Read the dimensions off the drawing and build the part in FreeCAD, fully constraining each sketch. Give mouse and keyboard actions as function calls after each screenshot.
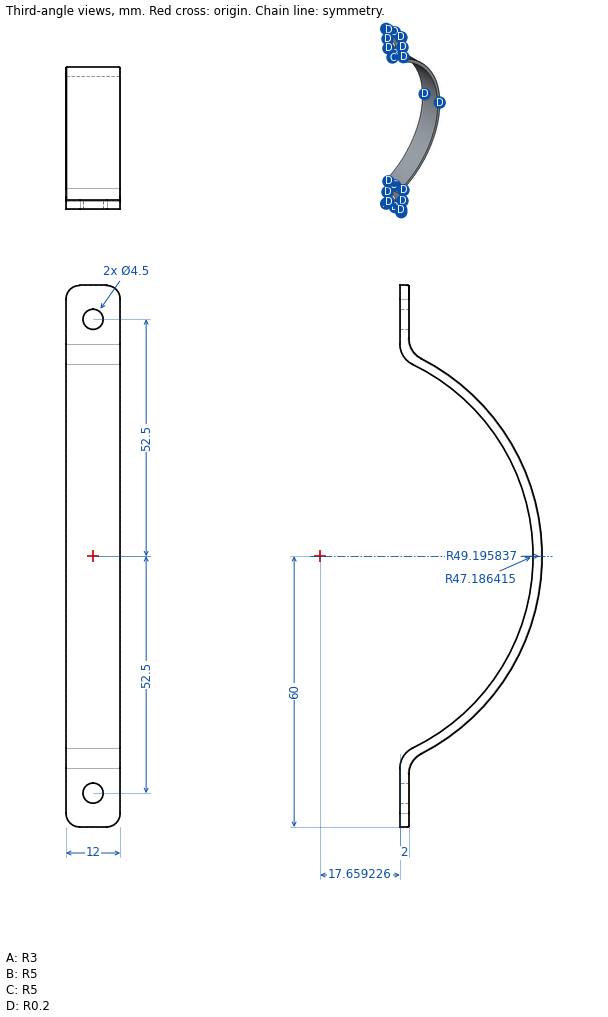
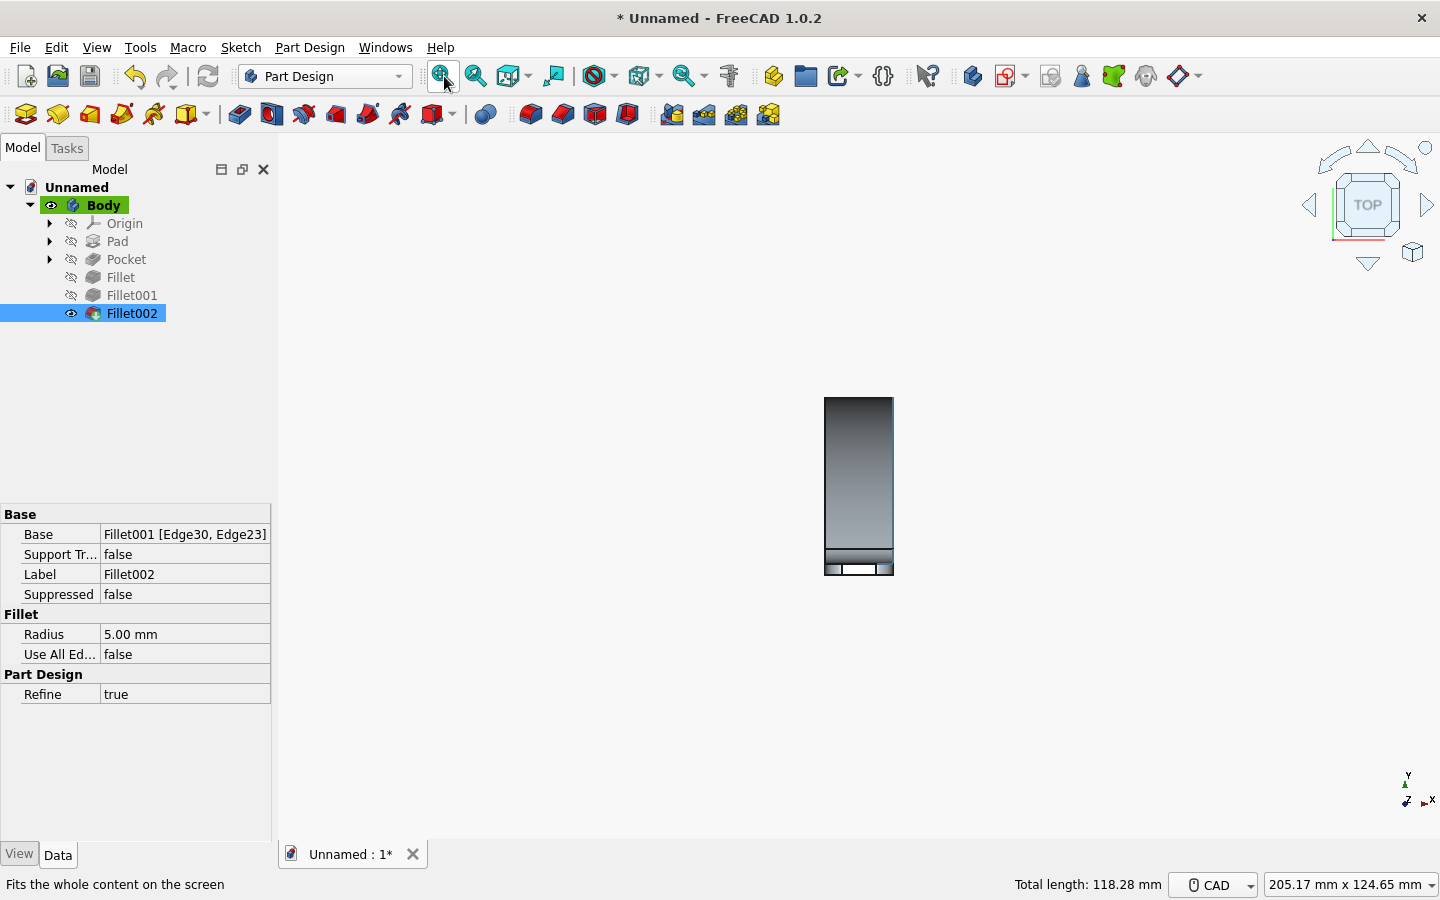
click(859, 563, ctrl)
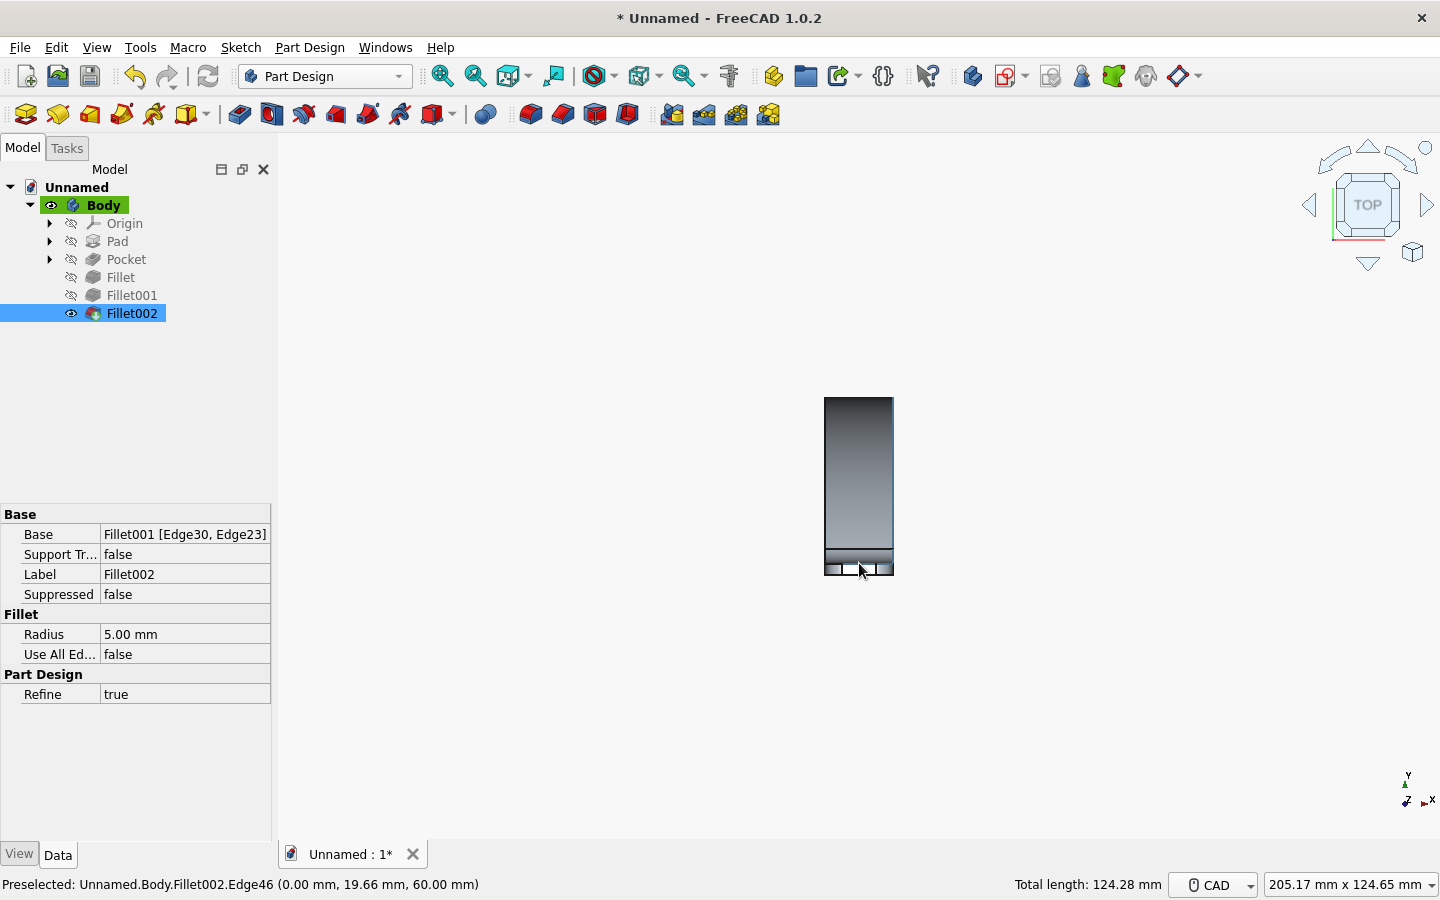
click(830, 563, ctrl)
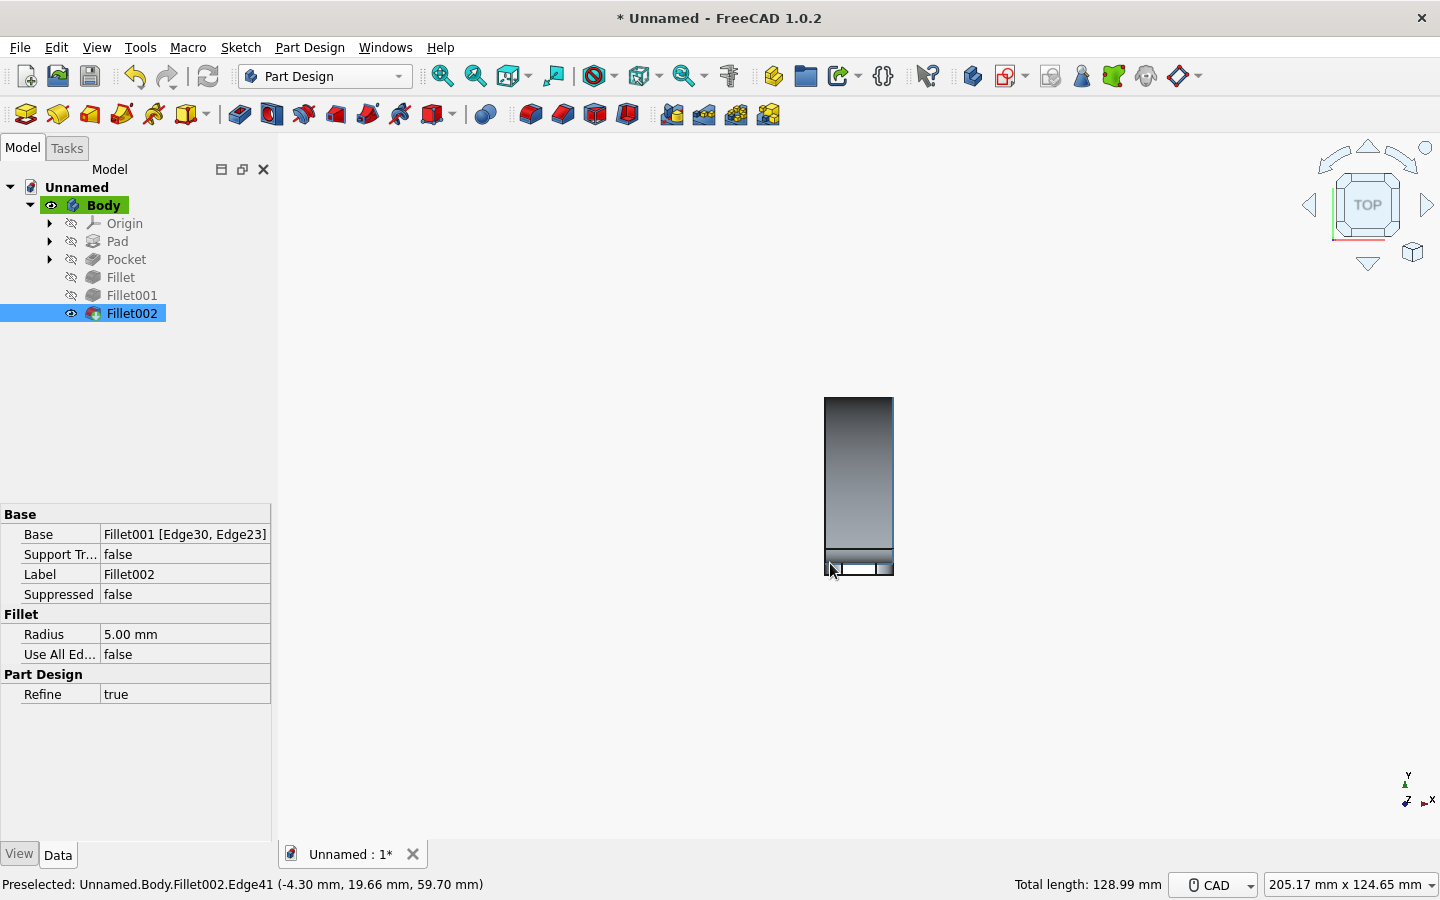
click(825, 402, ctrl)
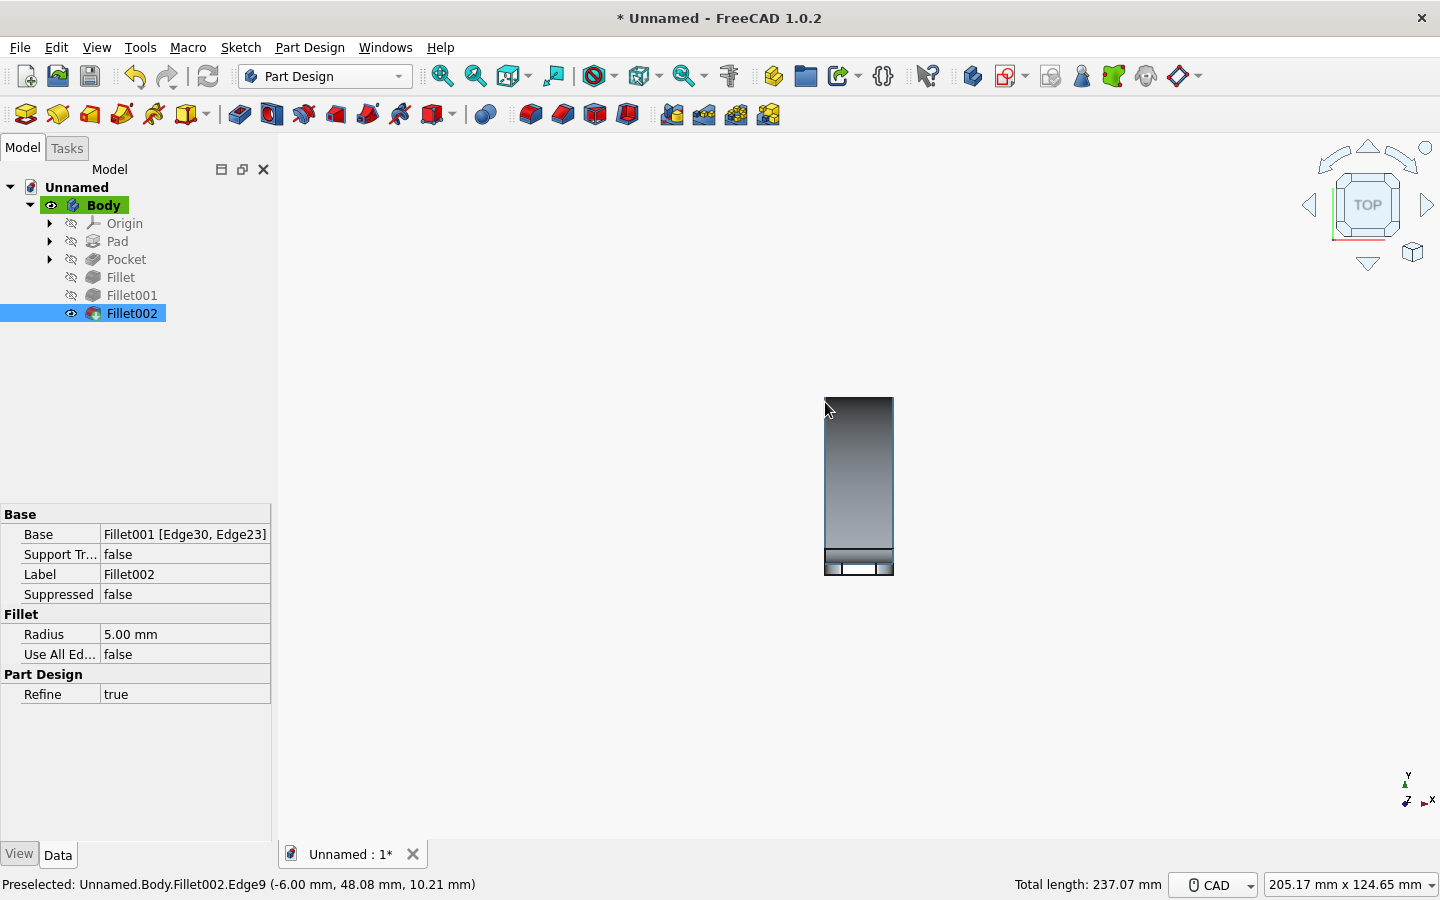
click(825, 555, ctrl)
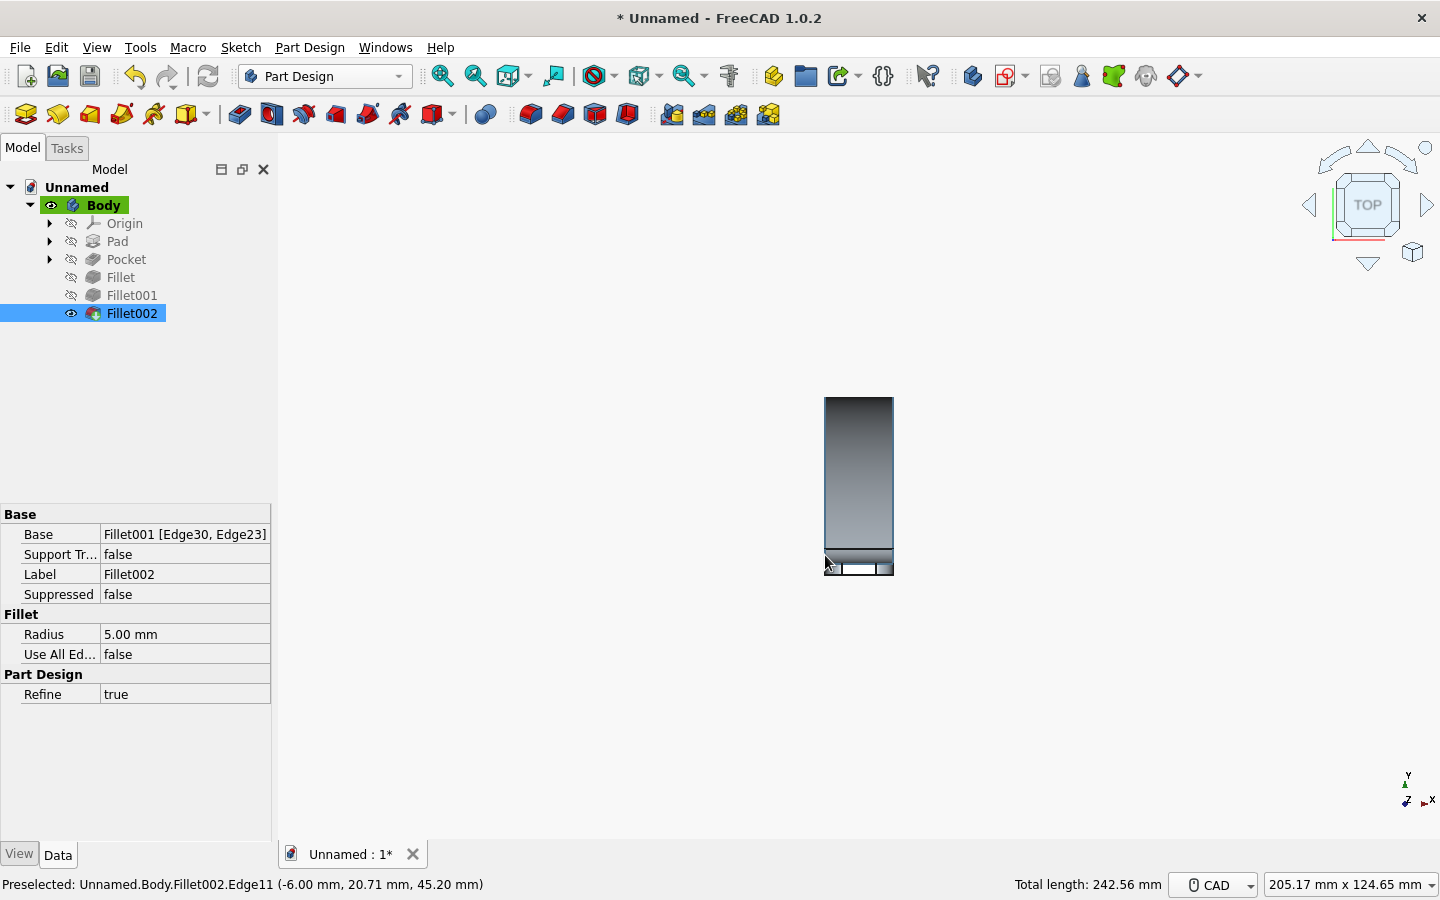
key(1)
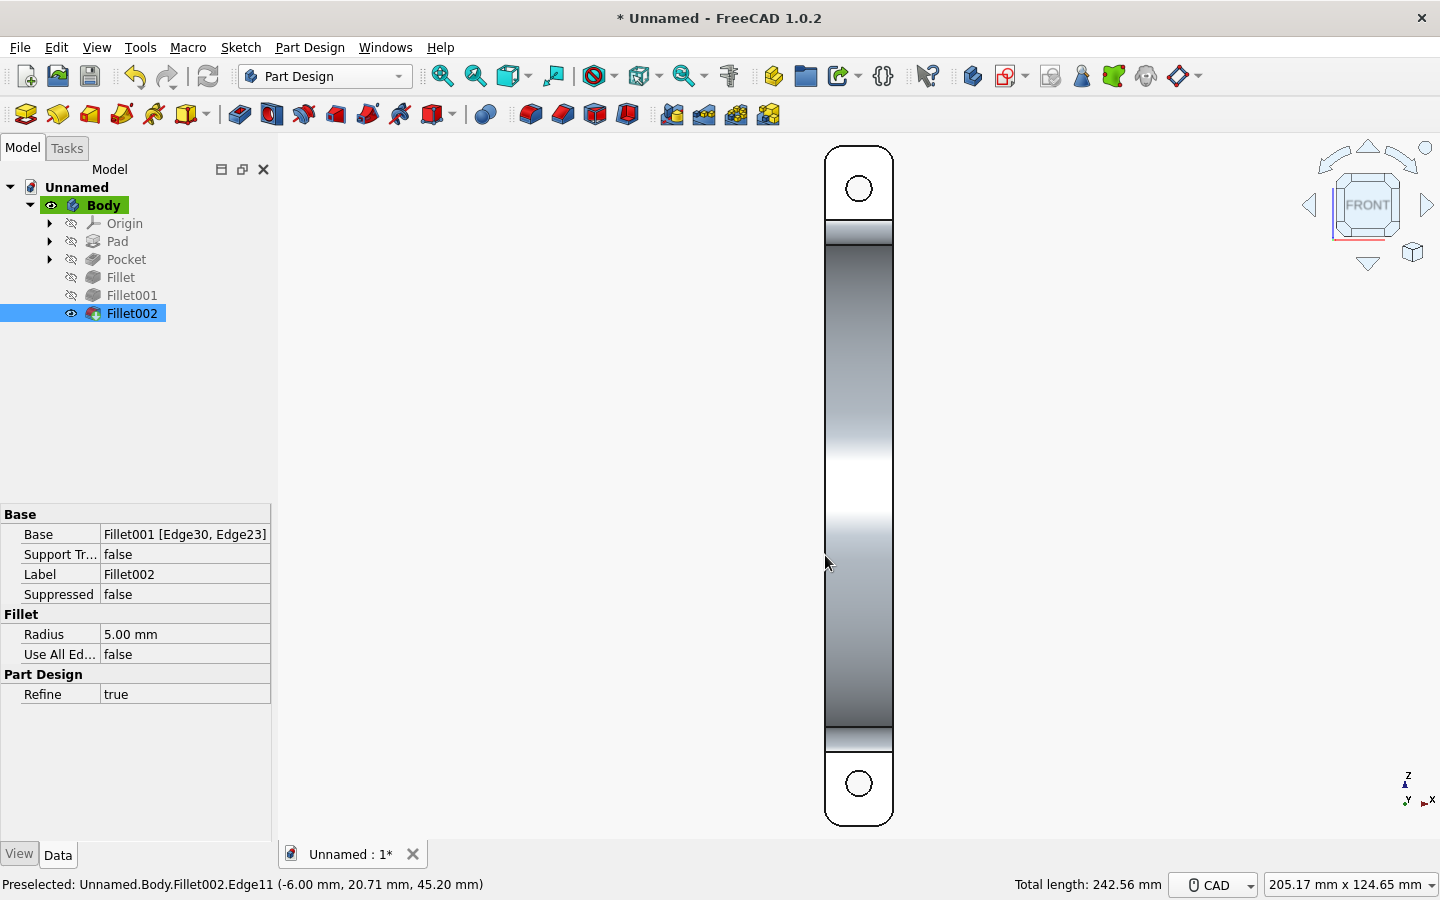
key(3)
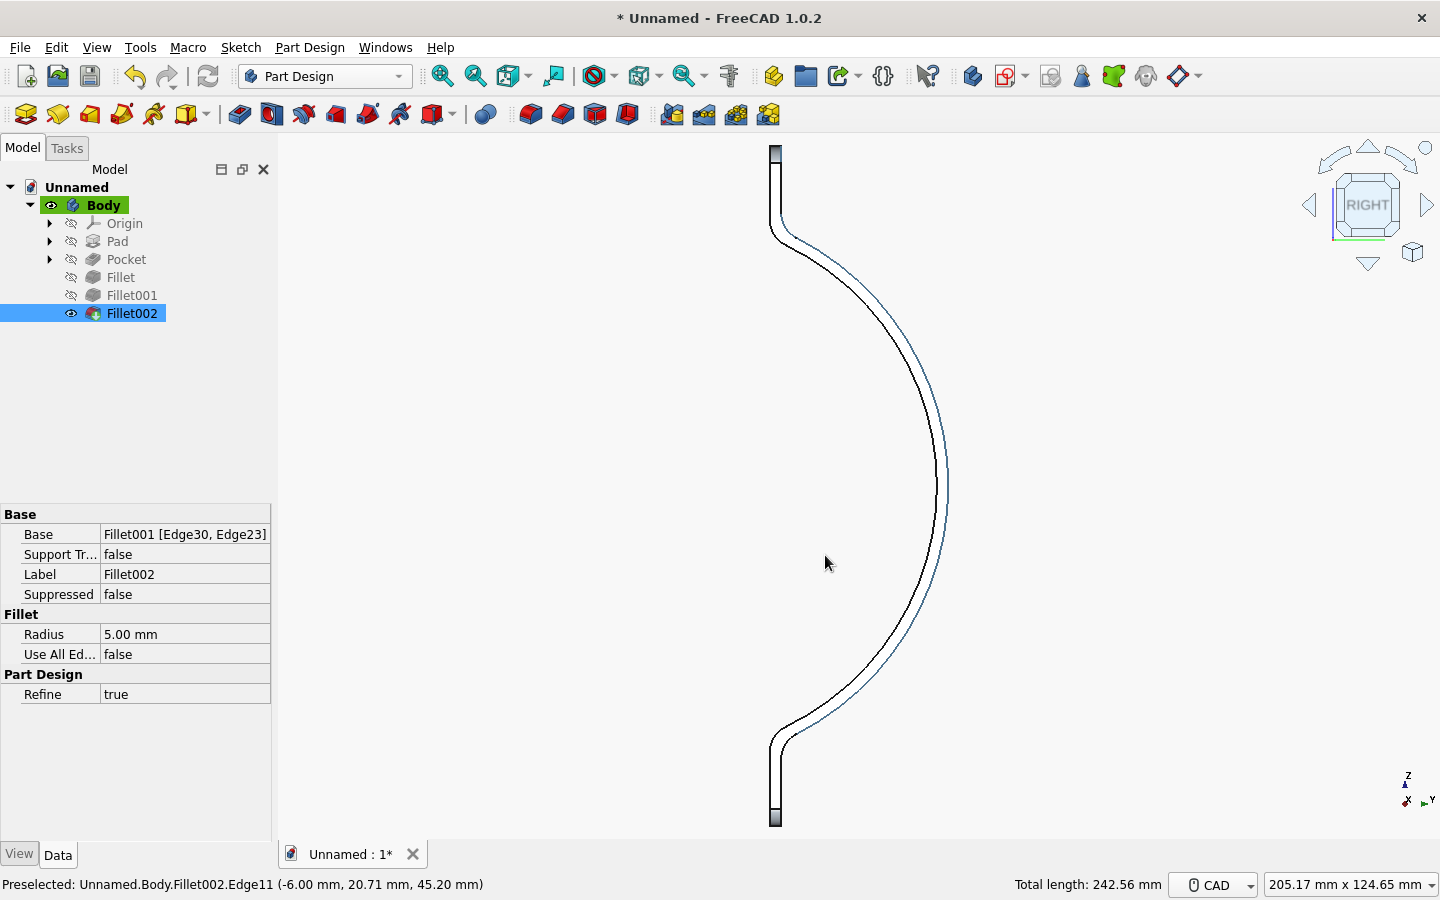
click(781, 783, ctrl)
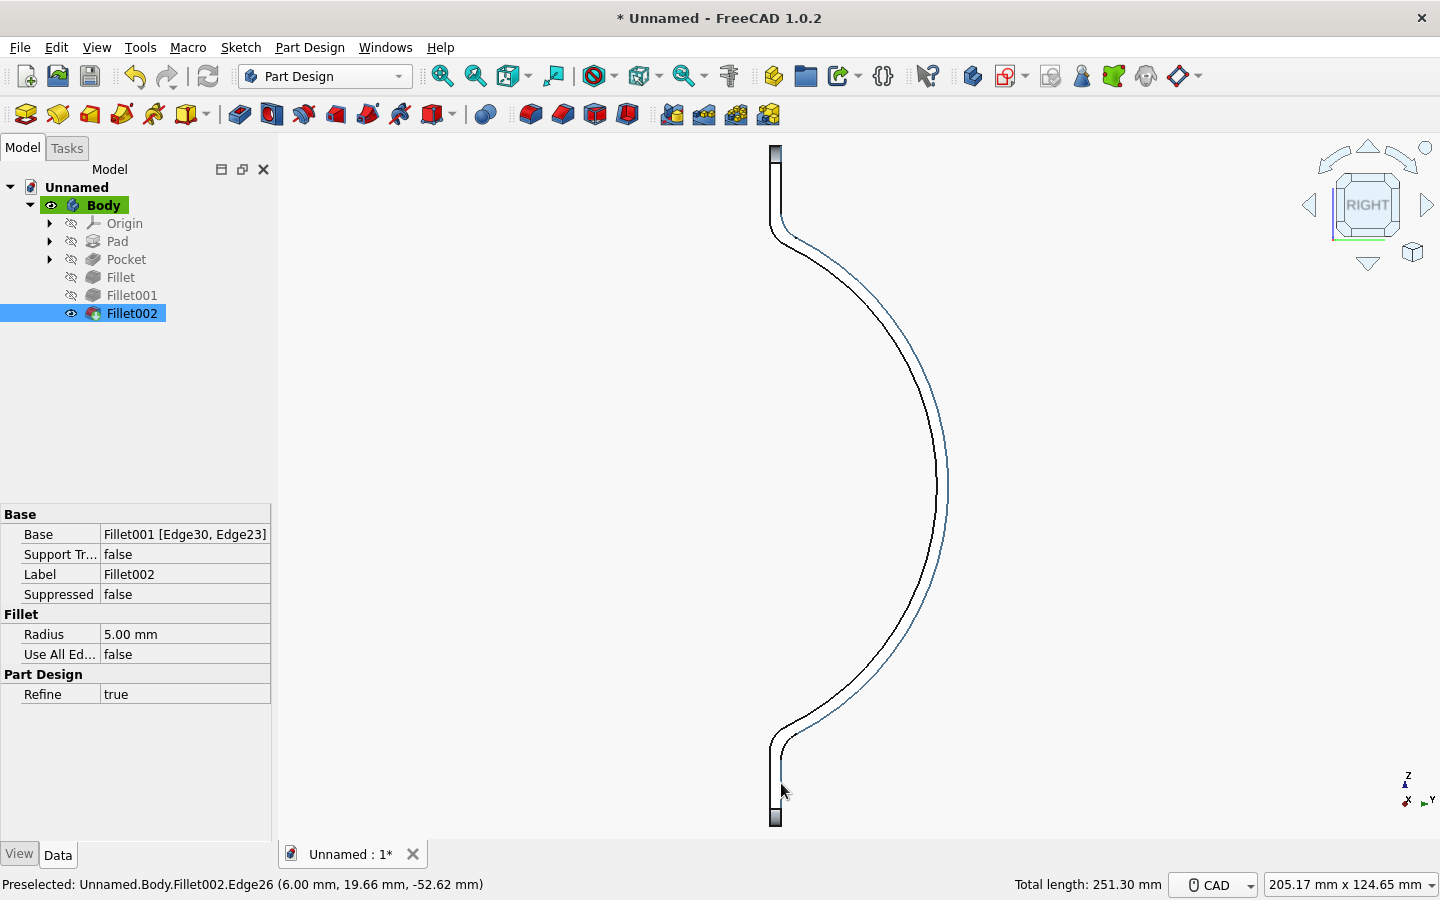
click(781, 187, ctrl)